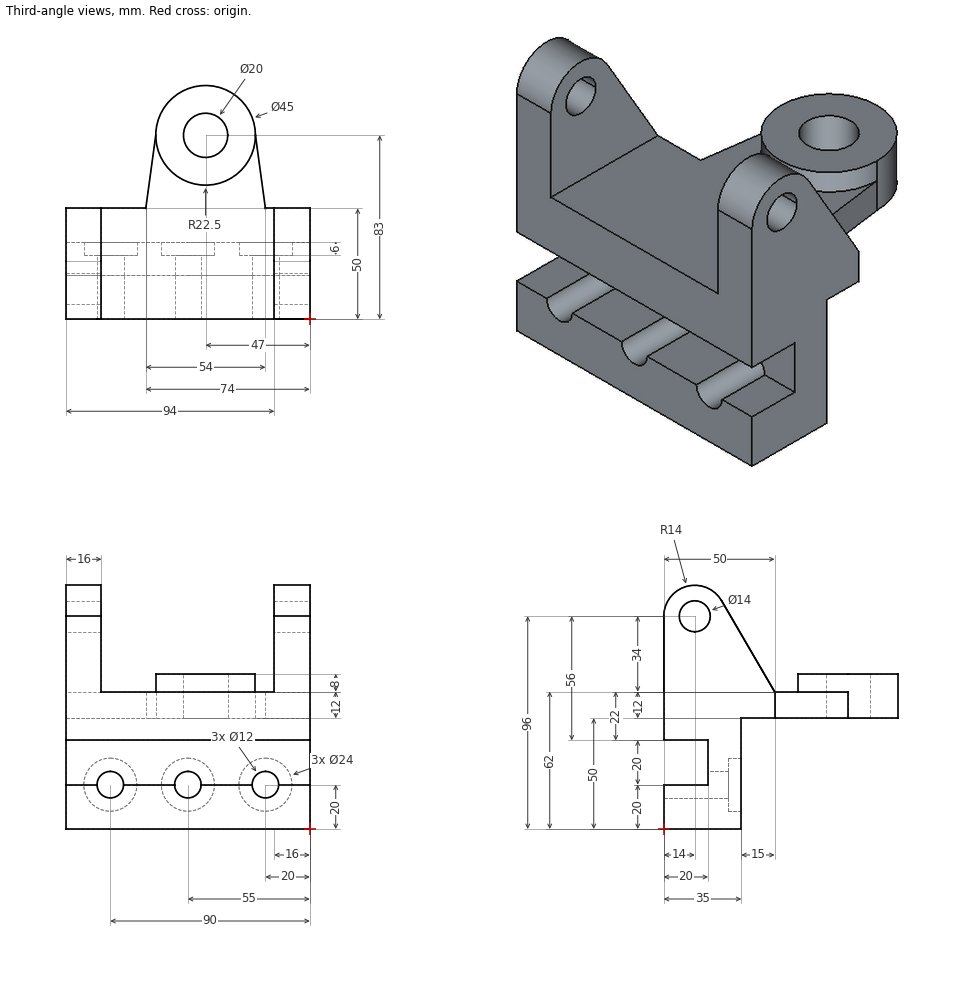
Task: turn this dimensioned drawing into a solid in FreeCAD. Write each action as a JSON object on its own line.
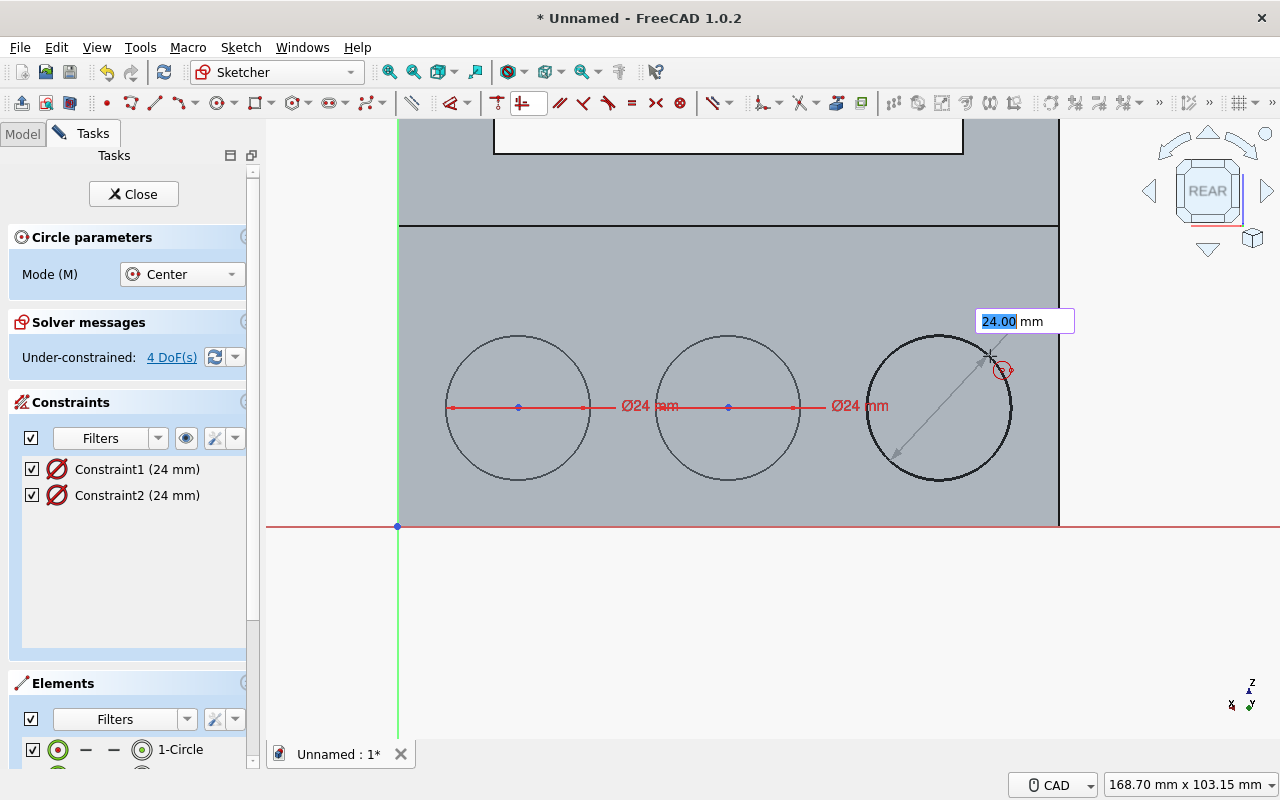
{"action": "type", "text": "24"}
{"action": "key", "text": "Return"}
{"action": "key", "text": "Escape"}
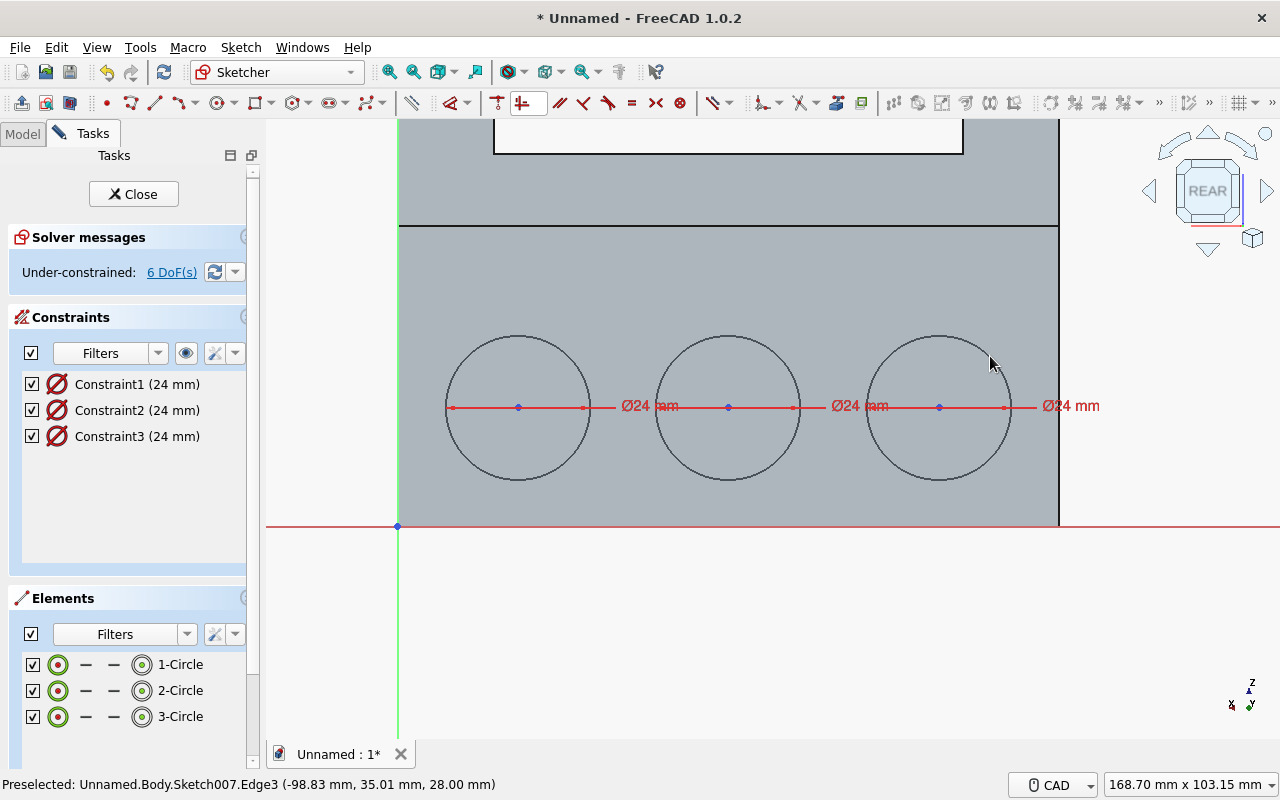
{"action": "left_click", "coordinate": [518, 408]}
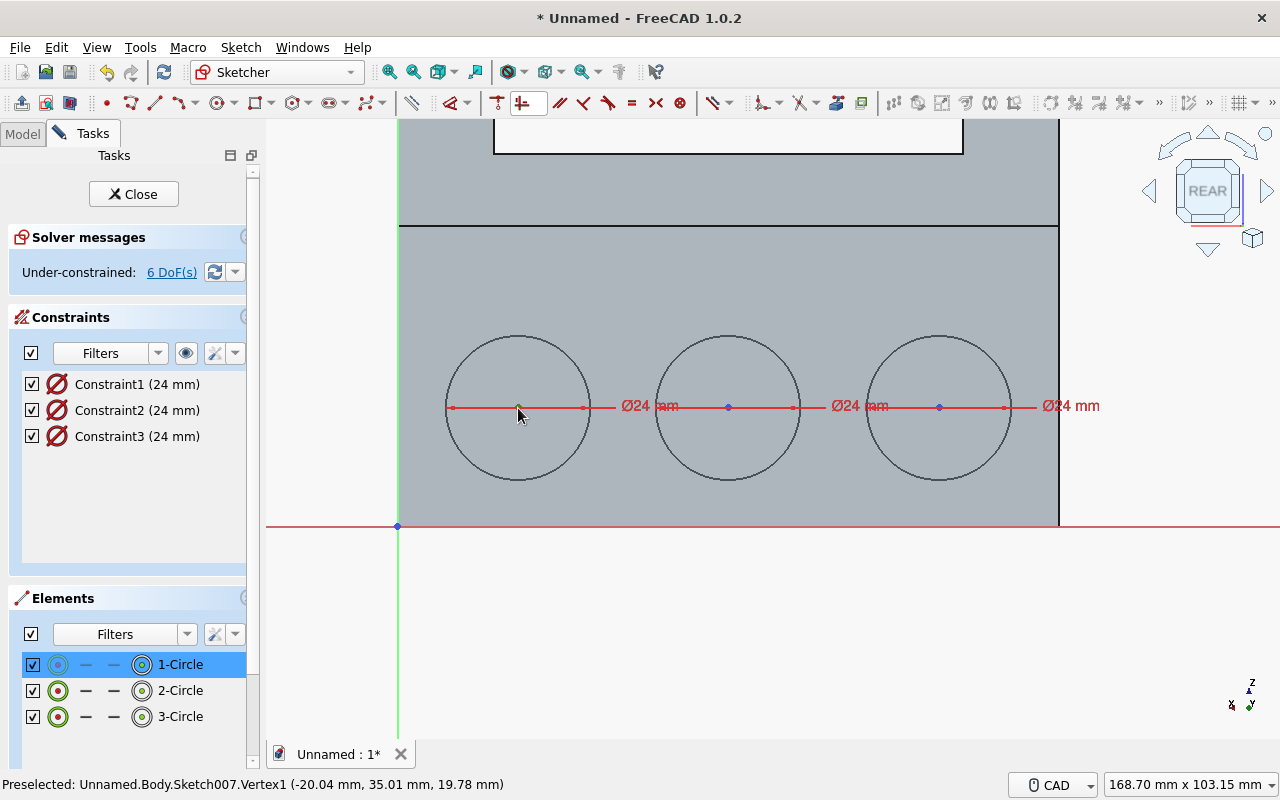
{"action": "left_click", "coordinate": [728, 408]}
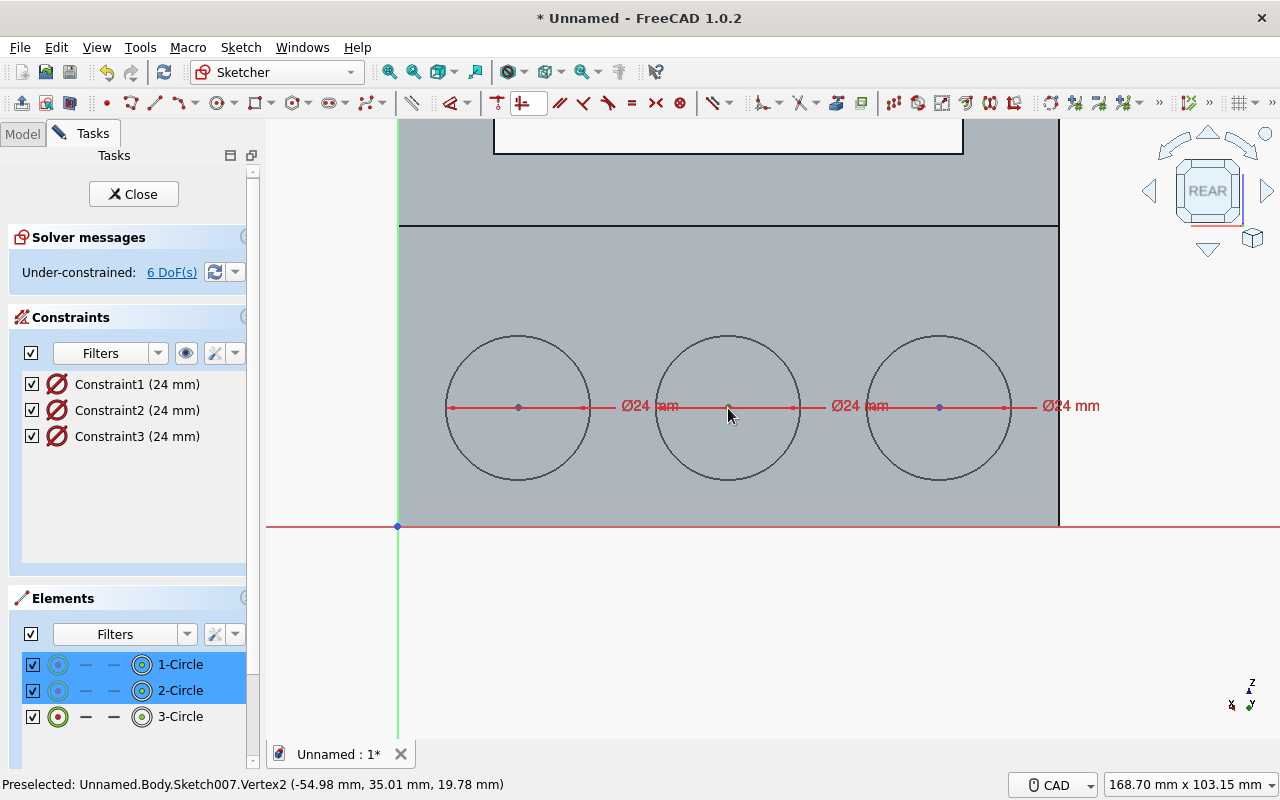
{"action": "left_click", "coordinate": [542, 104]}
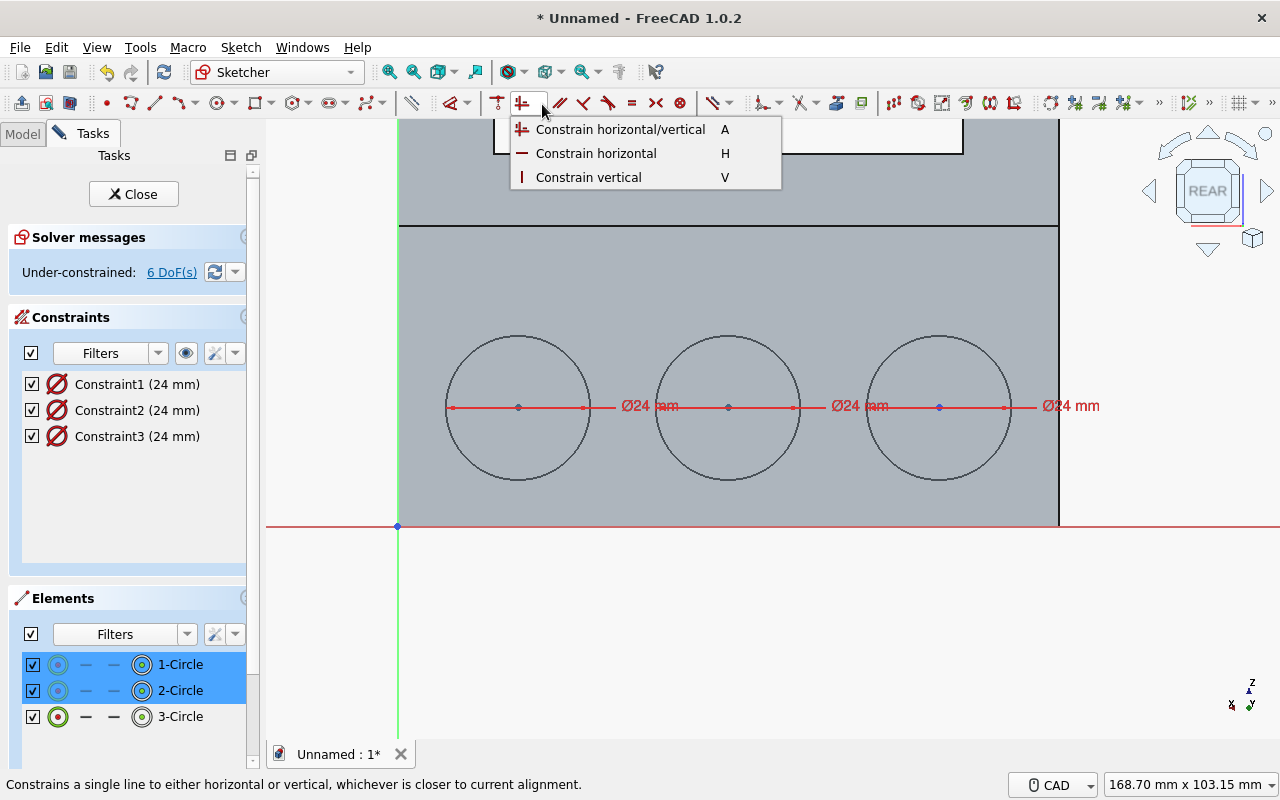
{"action": "left_click", "coordinate": [646, 153]}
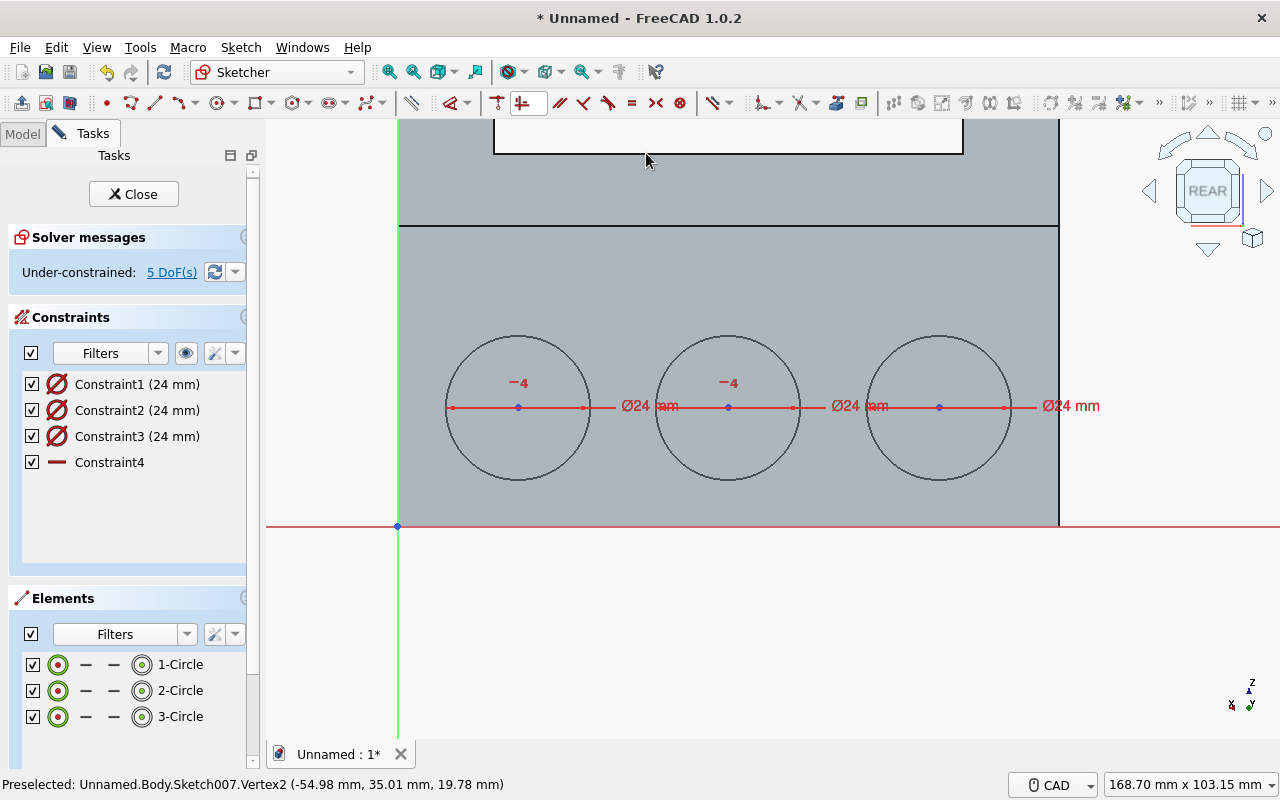
{"action": "left_click", "coordinate": [728, 408]}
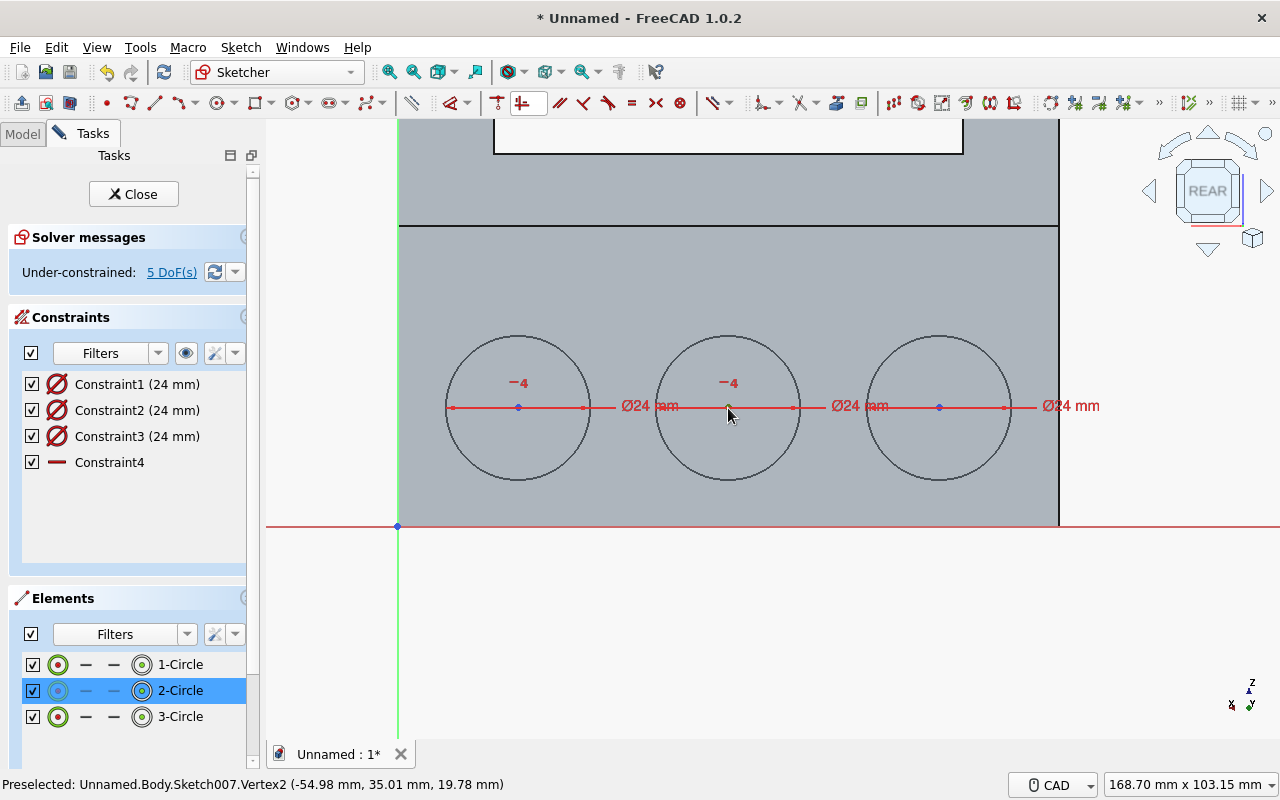
{"action": "left_click", "coordinate": [939, 408]}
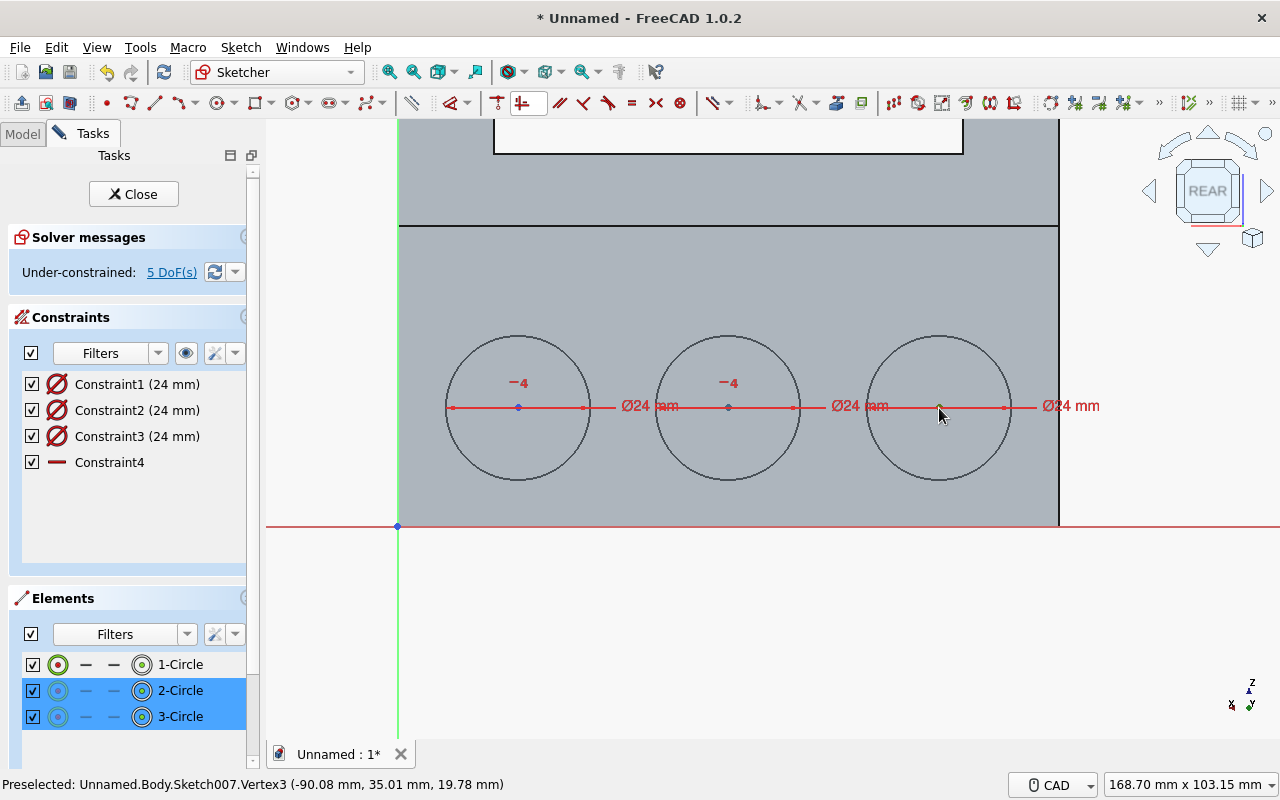
{"action": "left_click", "coordinate": [542, 104]}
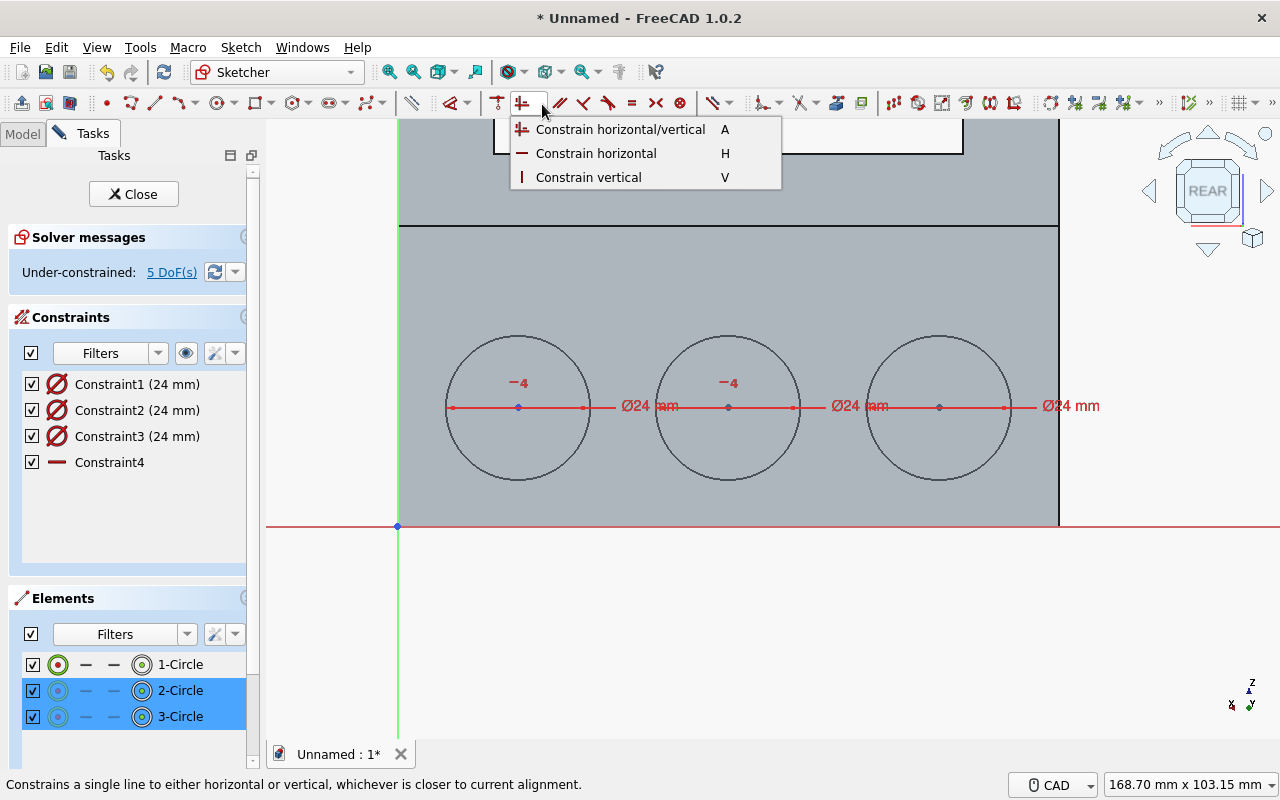
{"action": "left_click", "coordinate": [646, 153]}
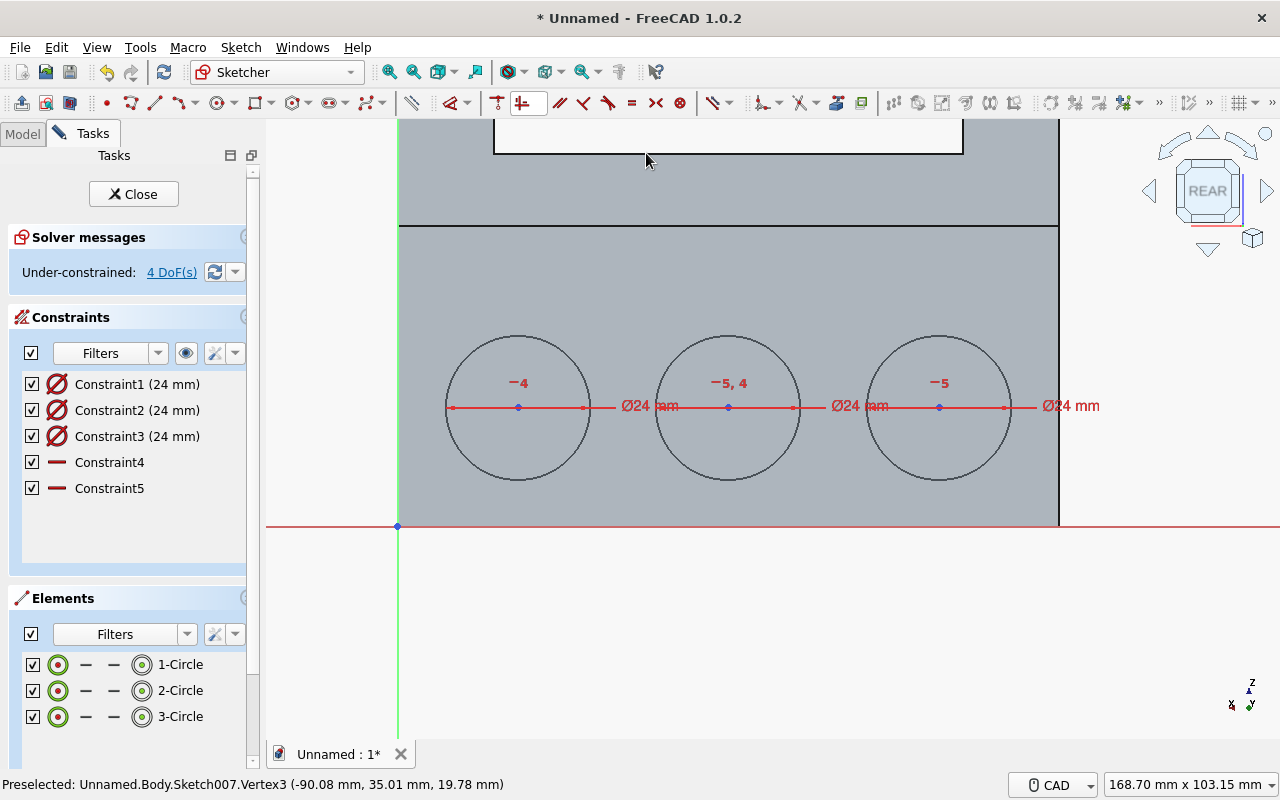
{"action": "left_click", "coordinate": [450, 104]}